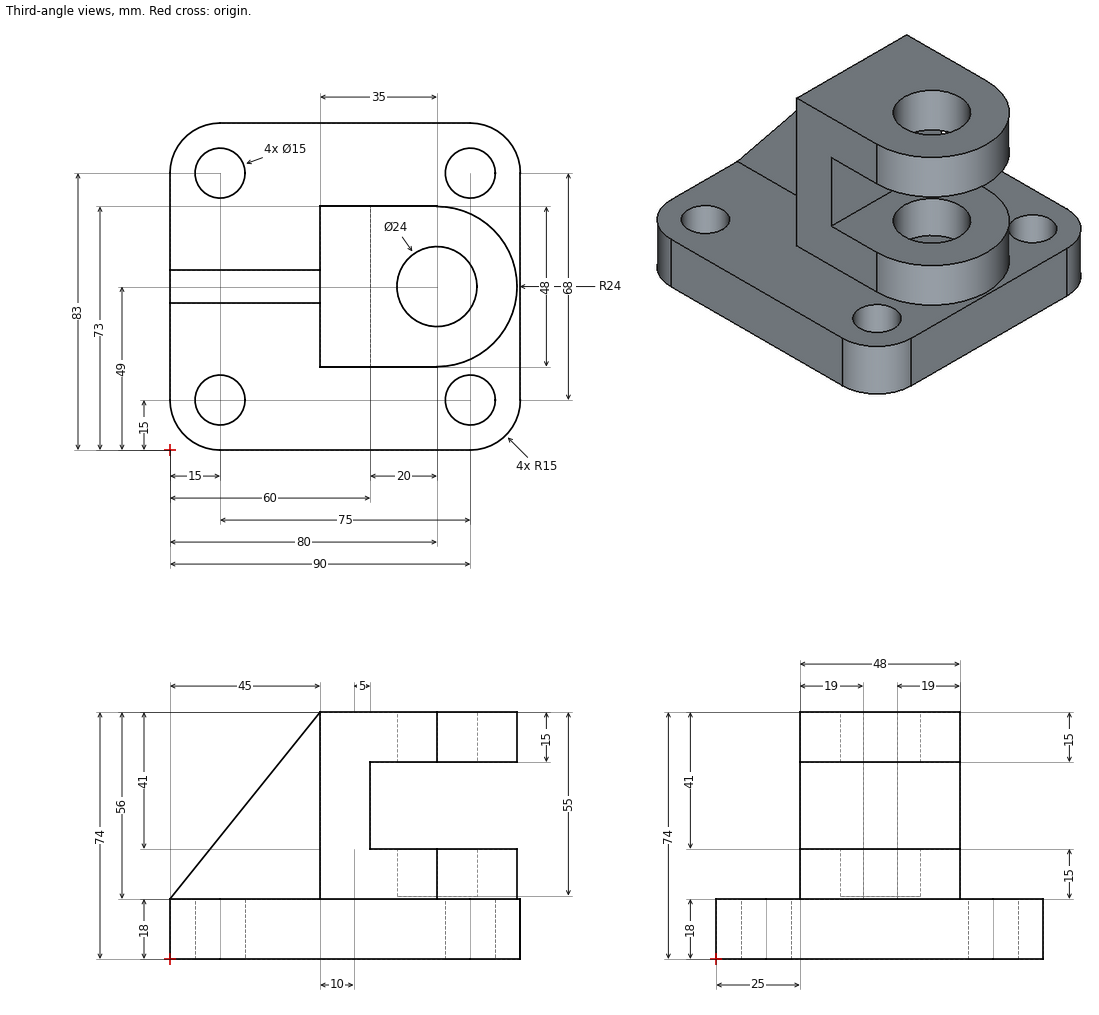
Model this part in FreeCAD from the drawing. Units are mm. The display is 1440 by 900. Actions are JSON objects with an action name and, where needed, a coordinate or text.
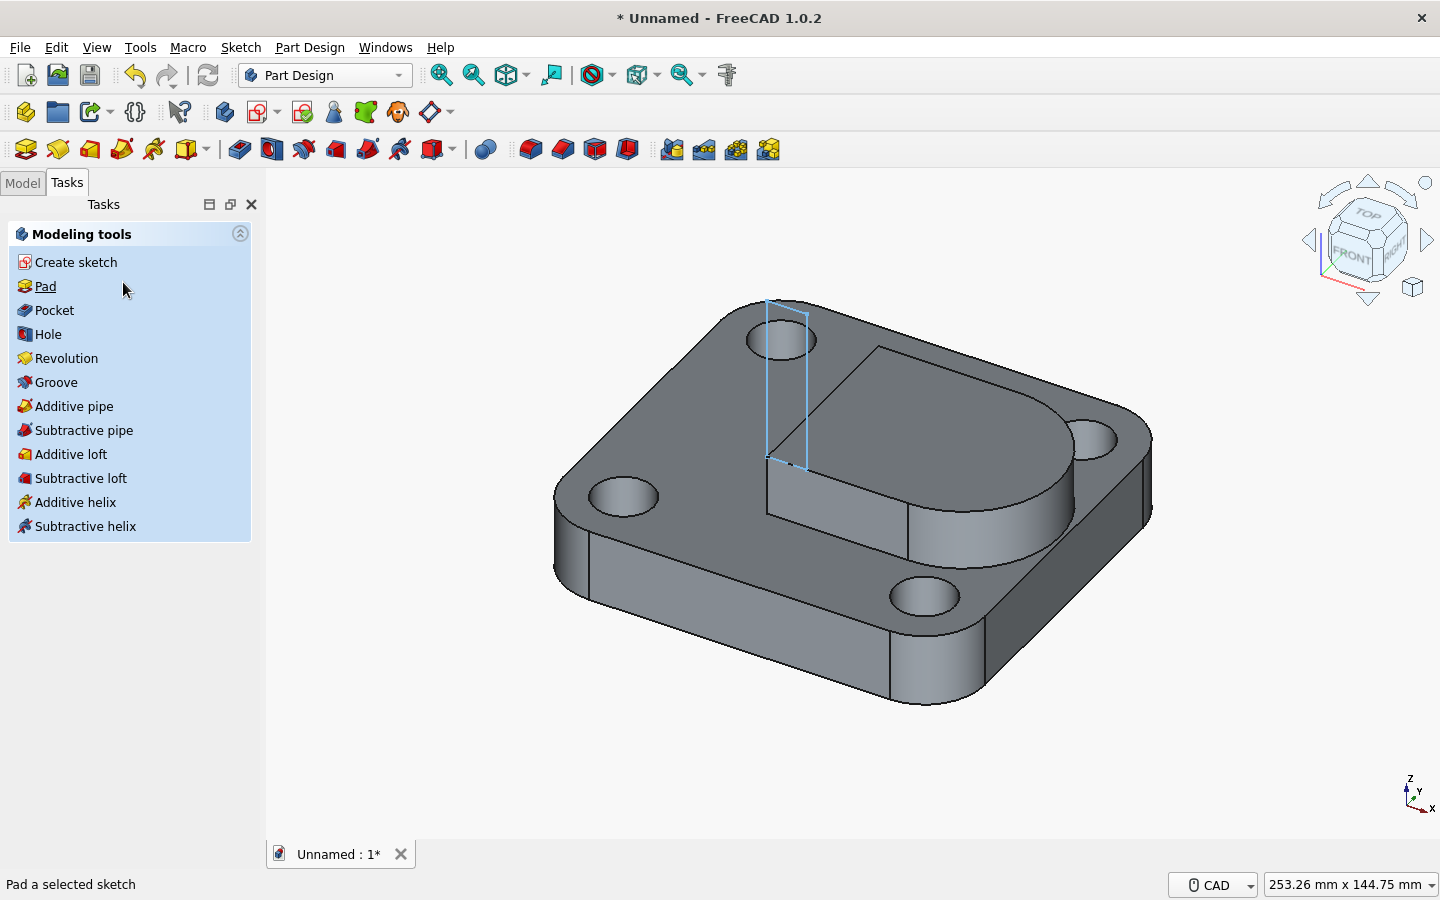
{"action": "left_click", "coordinate": [26, 150]}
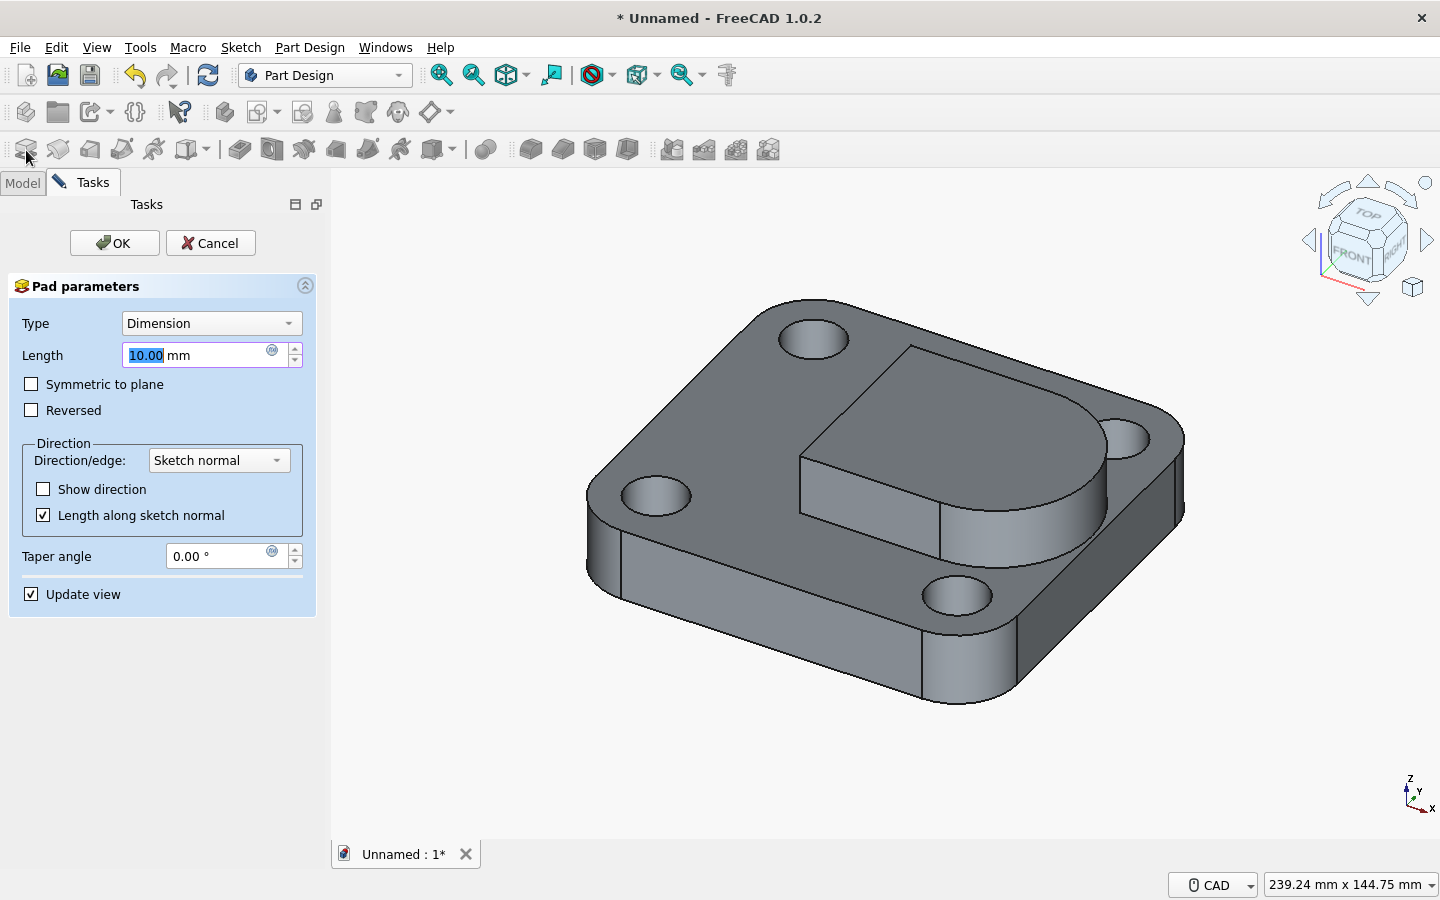
{"action": "type", "text": "48"}
{"action": "key", "text": "Tab"}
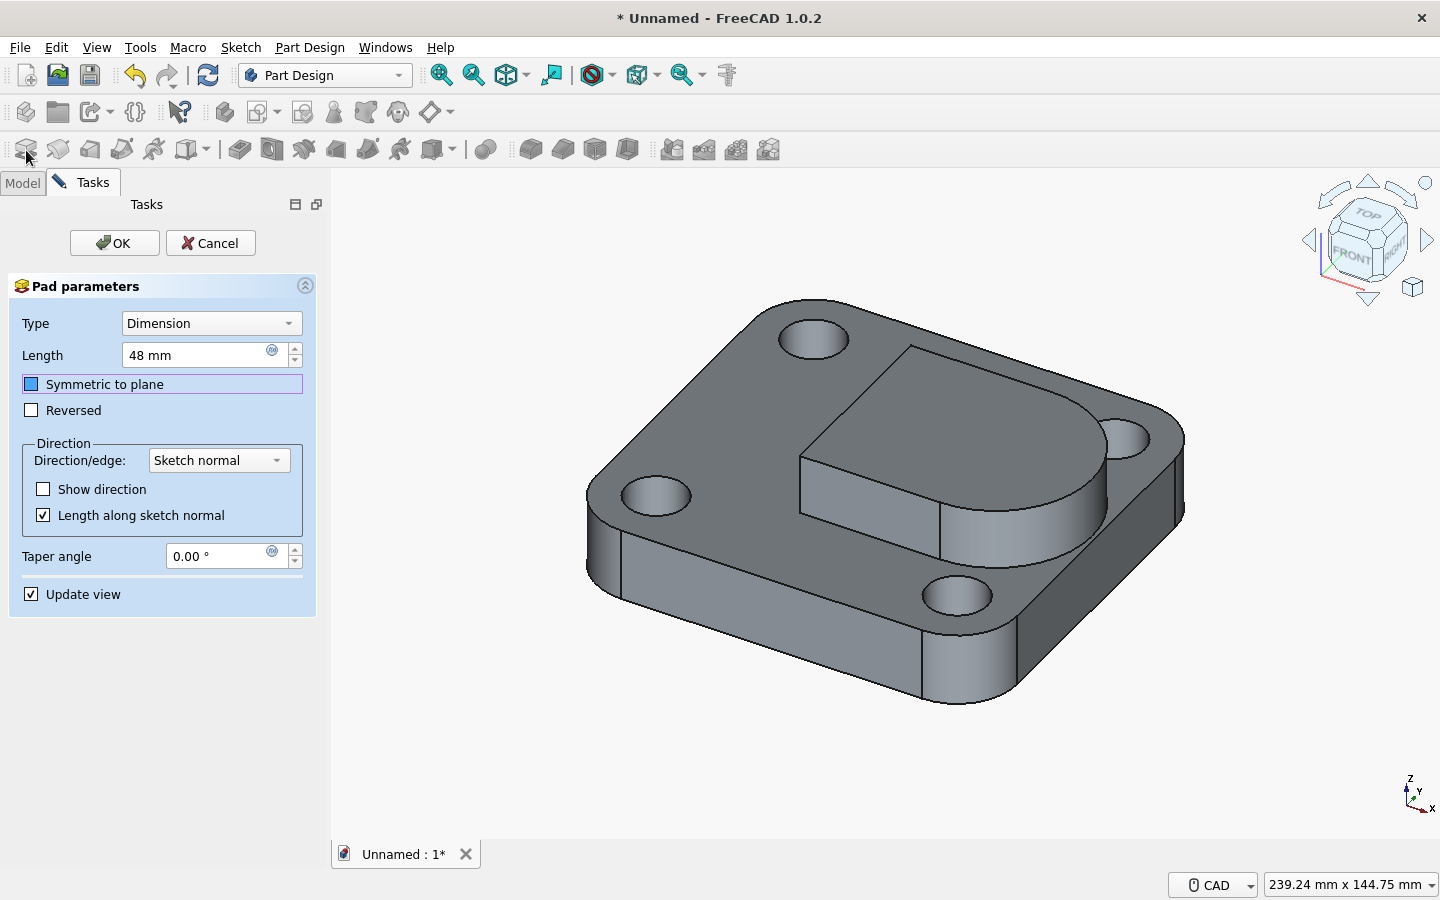
{"action": "left_click", "coordinate": [30, 410]}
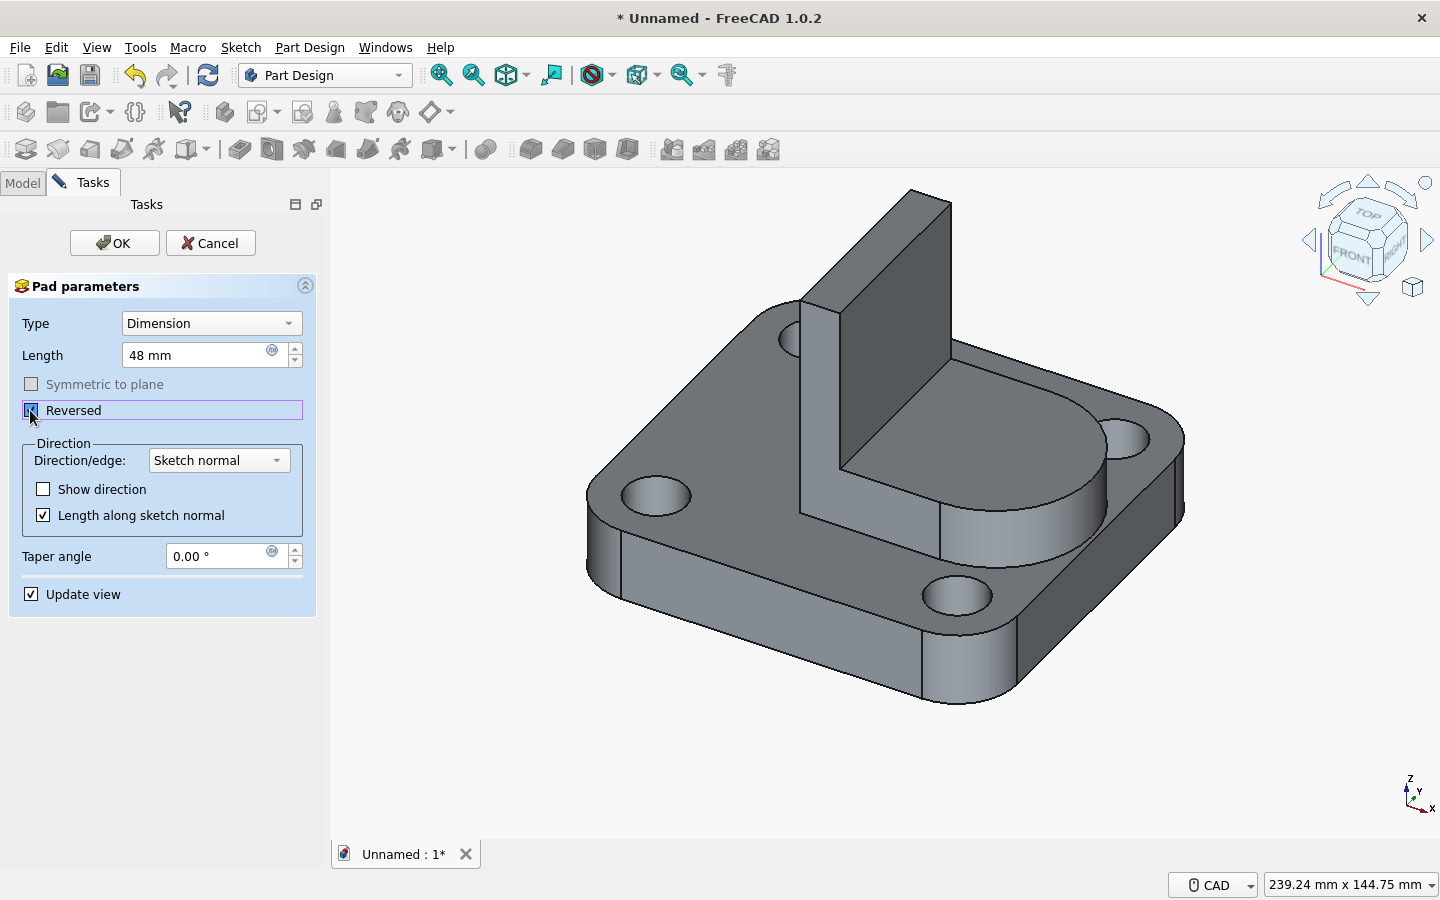
{"action": "left_click", "coordinate": [115, 243]}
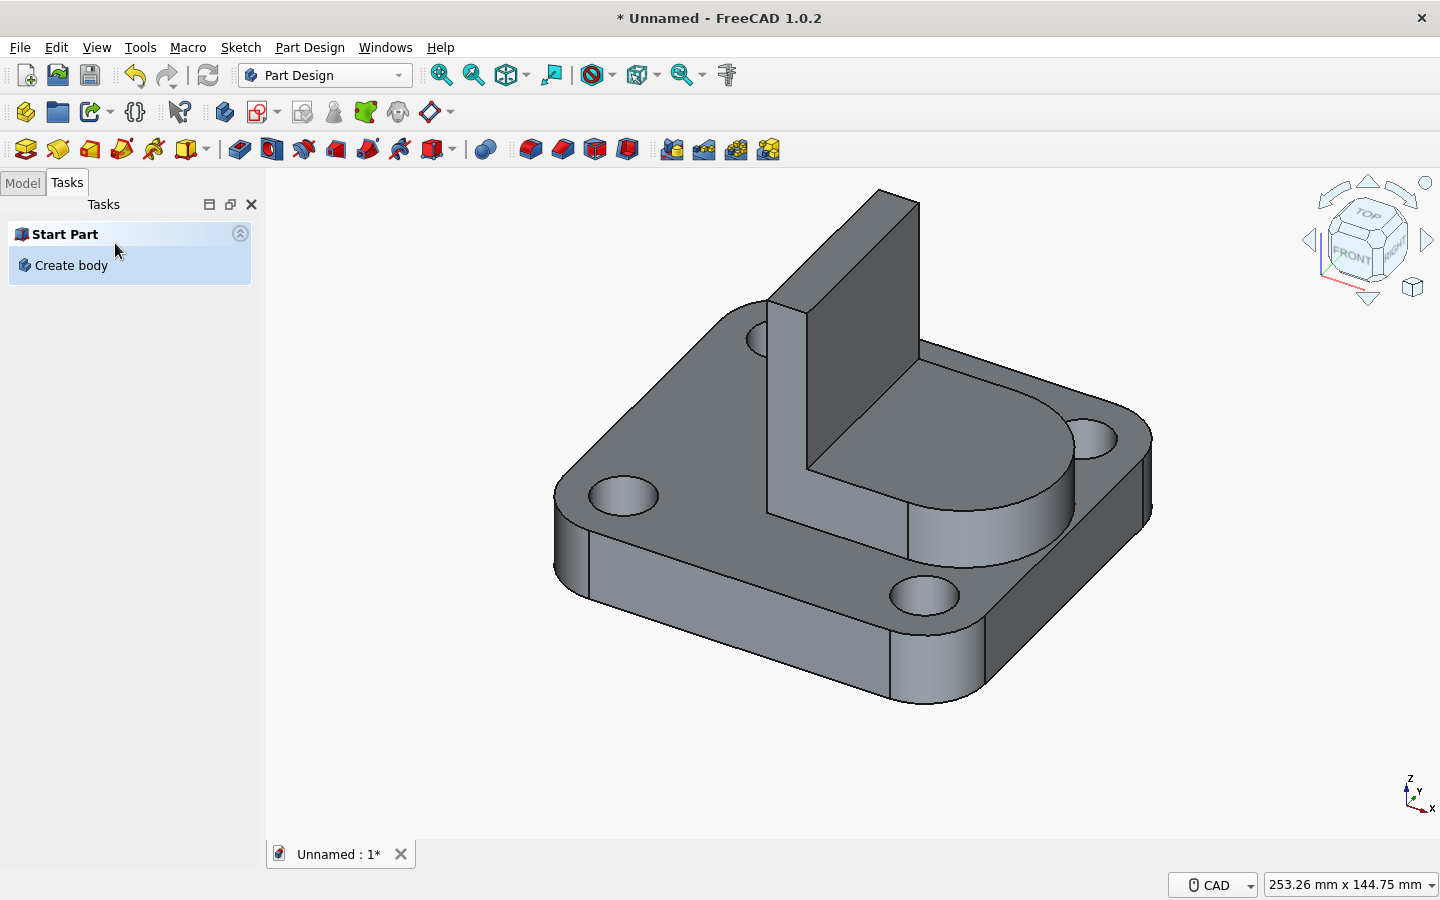
{"action": "left_click", "coordinate": [442, 76]}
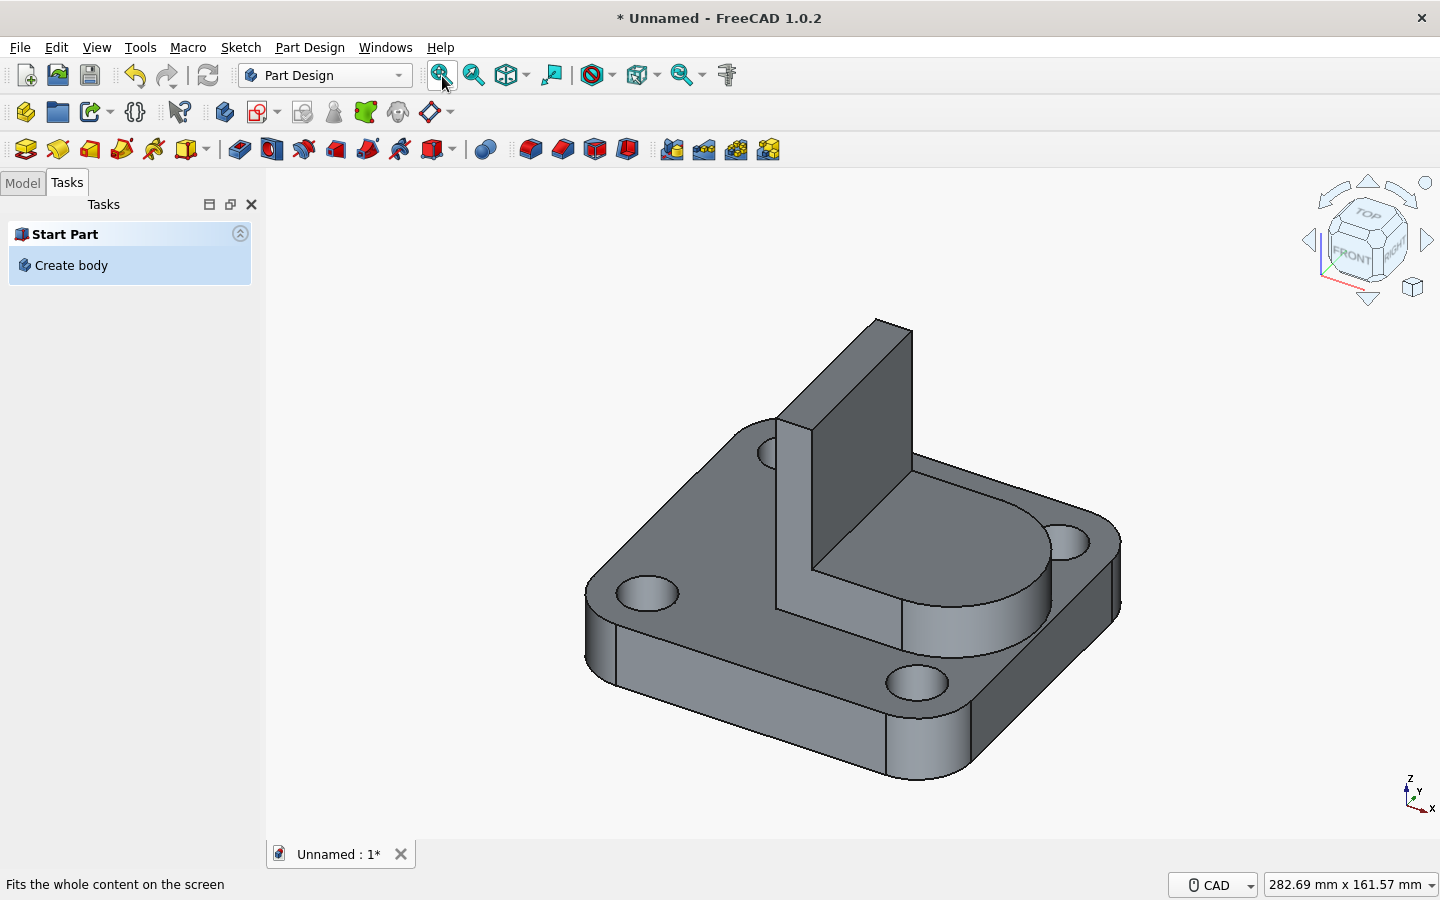
{"action": "left_click", "coordinate": [862, 449]}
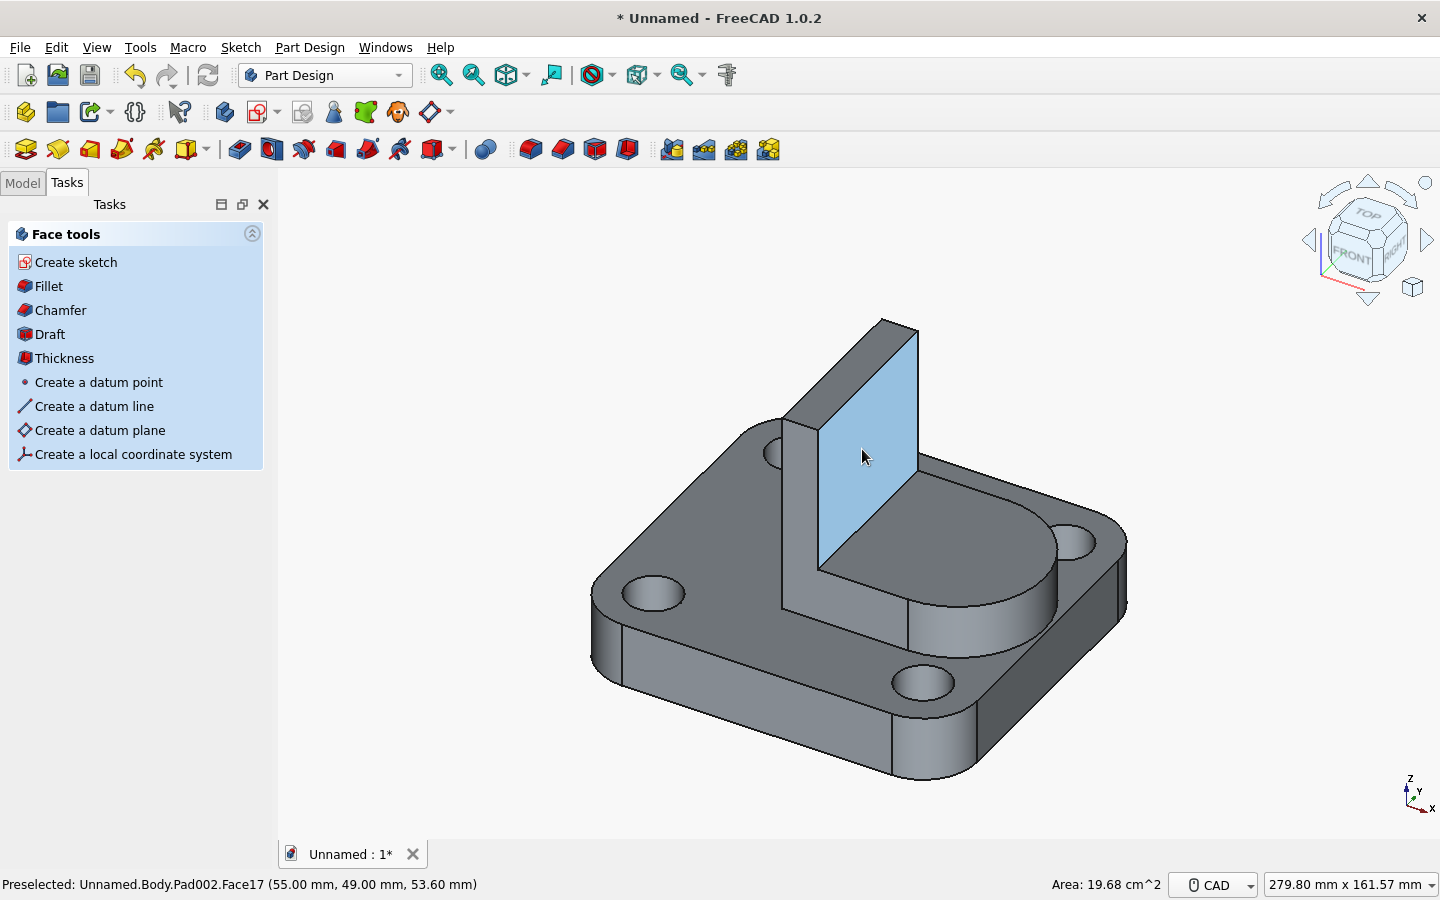
{"action": "left_click", "coordinate": [258, 112]}